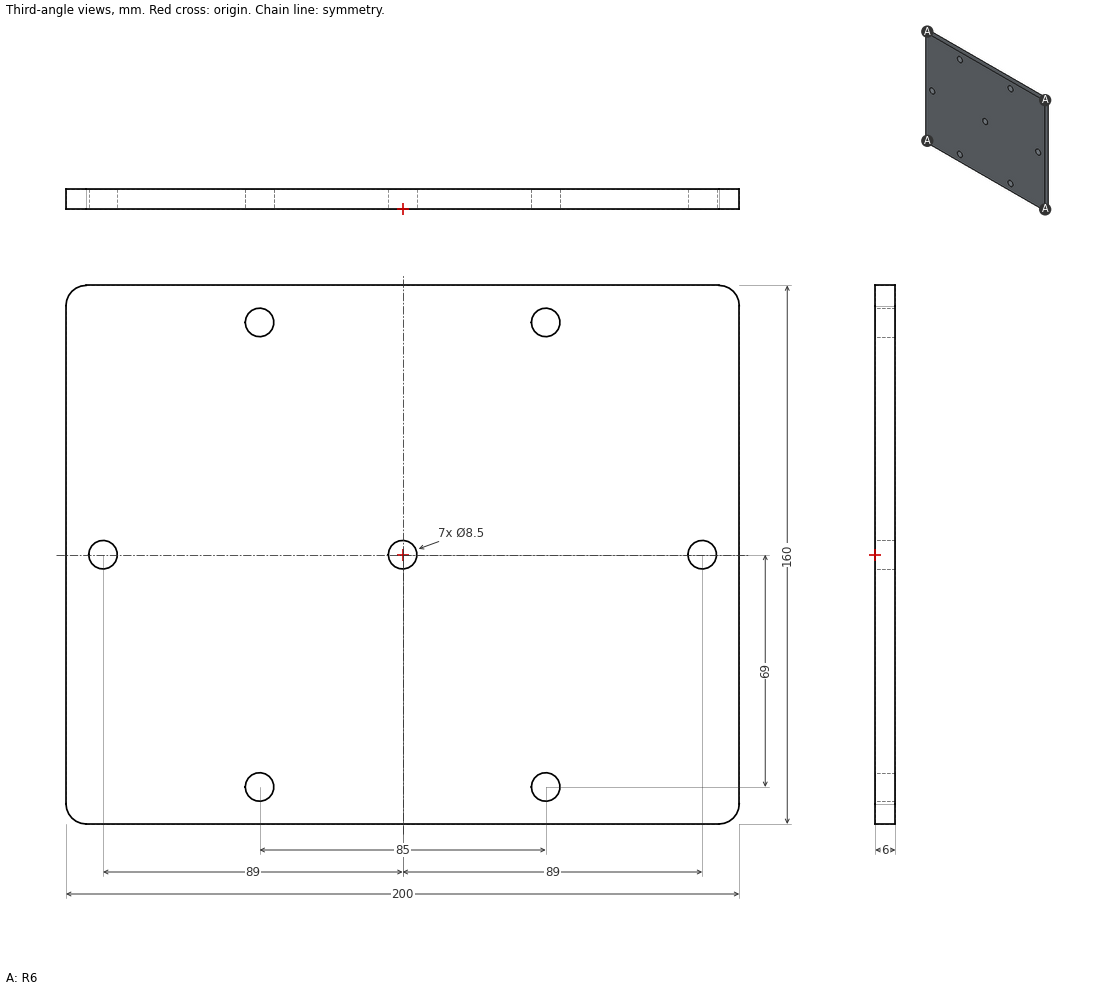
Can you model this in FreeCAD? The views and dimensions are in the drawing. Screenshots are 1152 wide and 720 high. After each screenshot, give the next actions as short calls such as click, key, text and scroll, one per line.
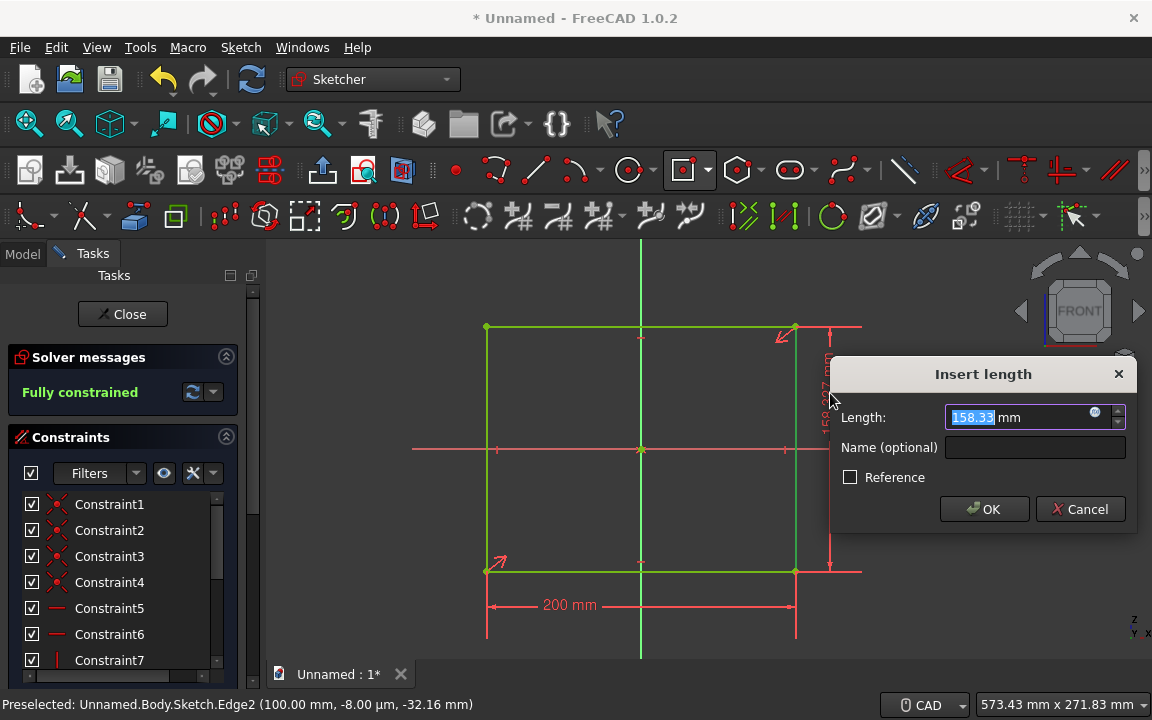
text(160)
key(Return)
key(Escape)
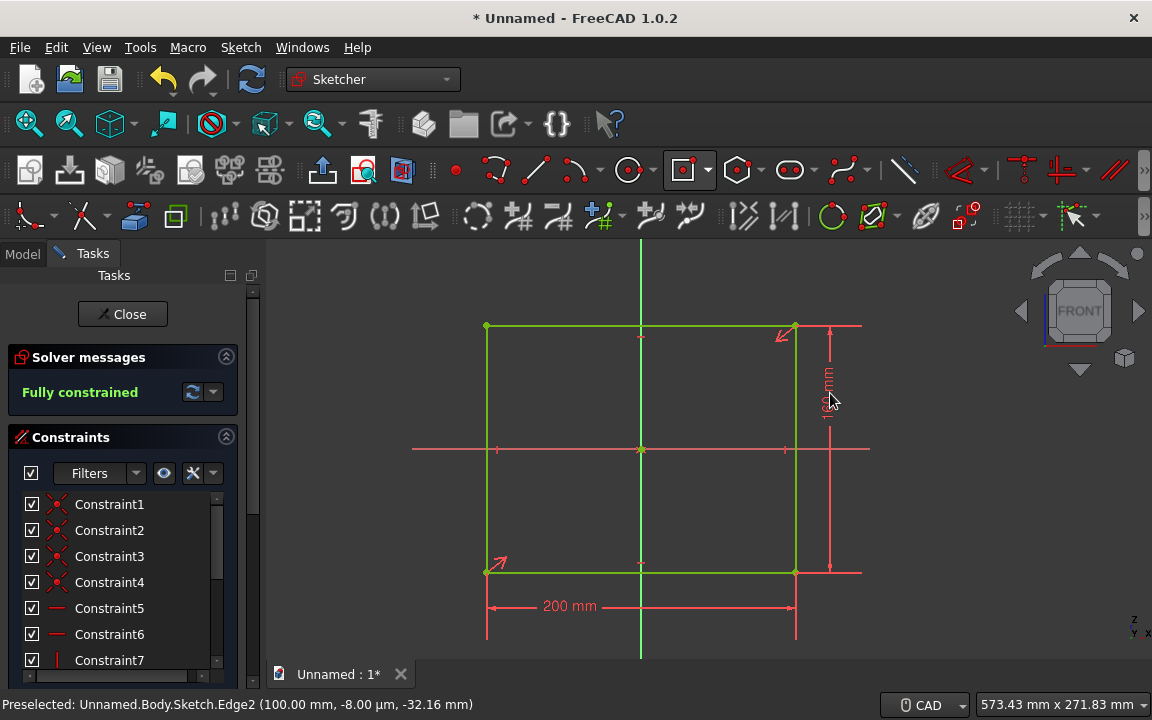
click(123, 314)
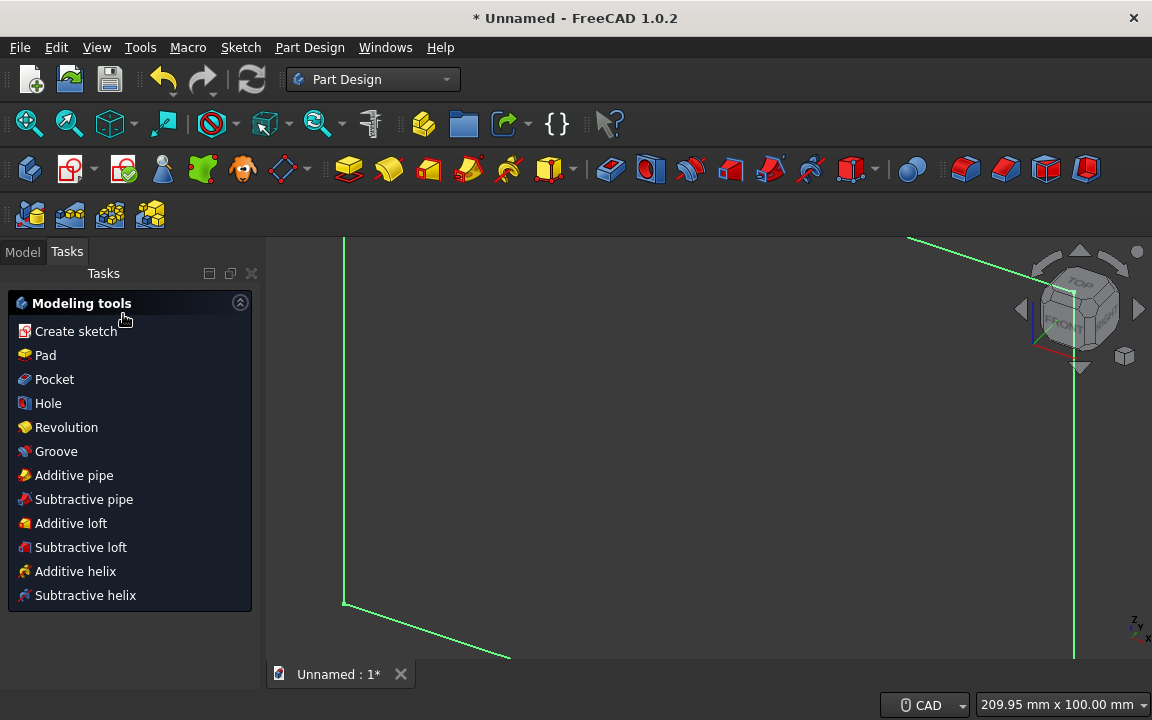
click(350, 170)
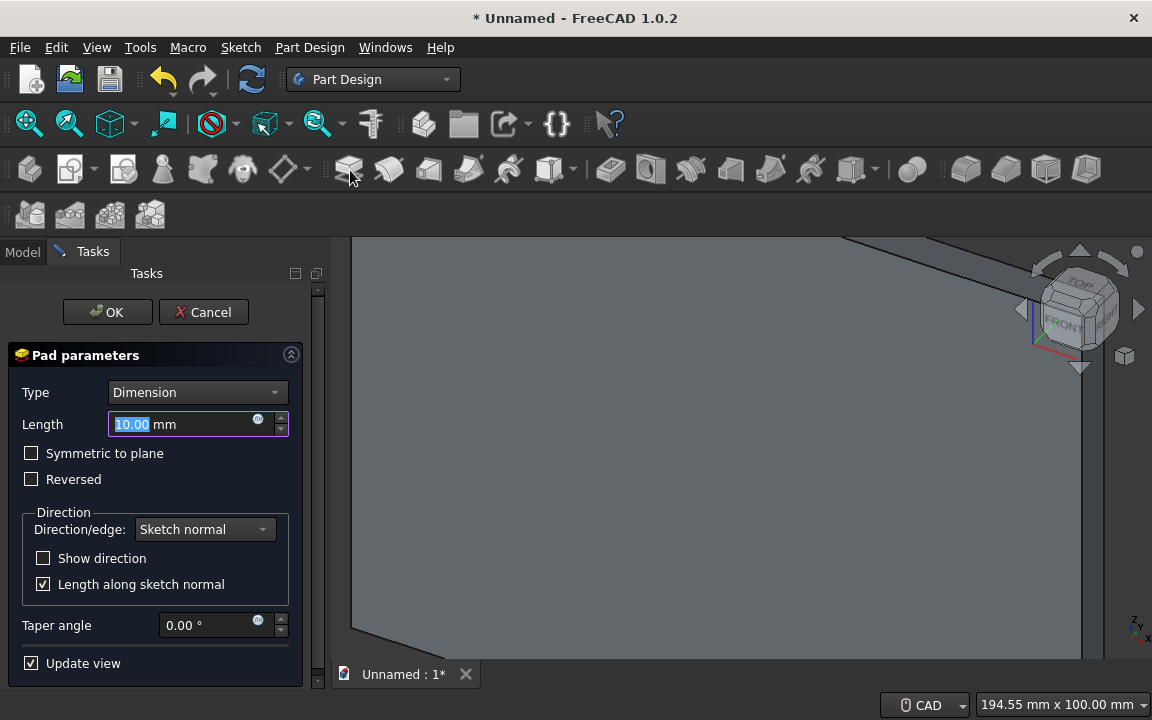
text(6)
key(Tab)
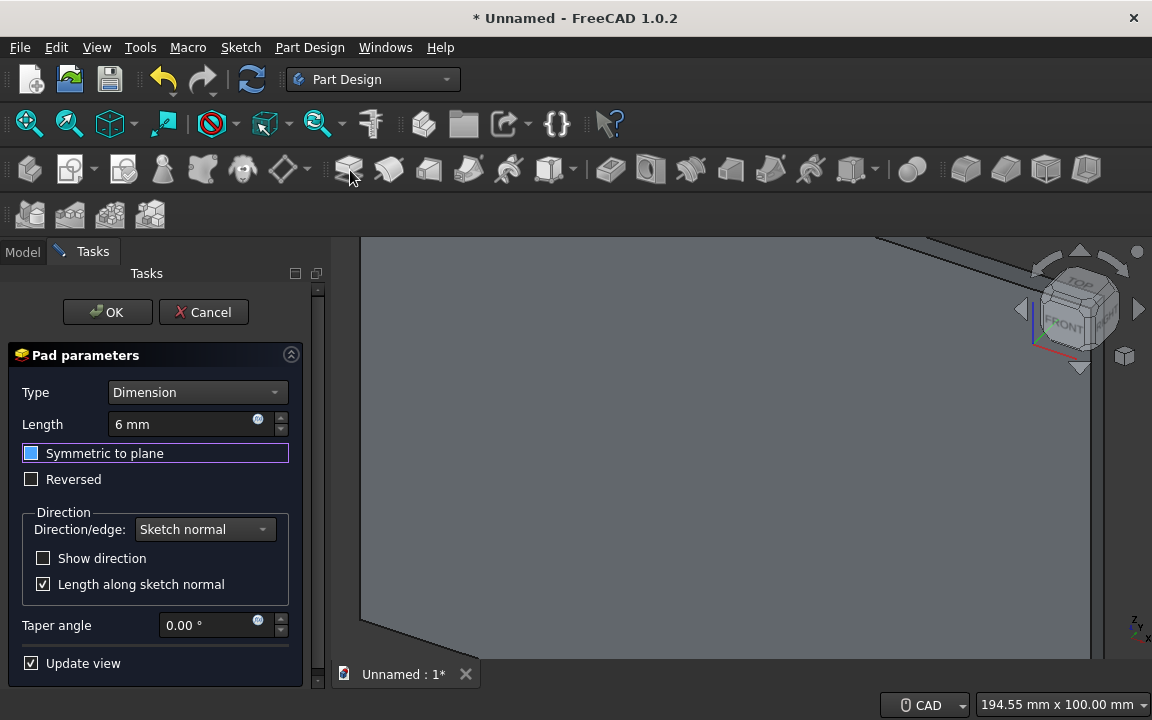
click(30, 479)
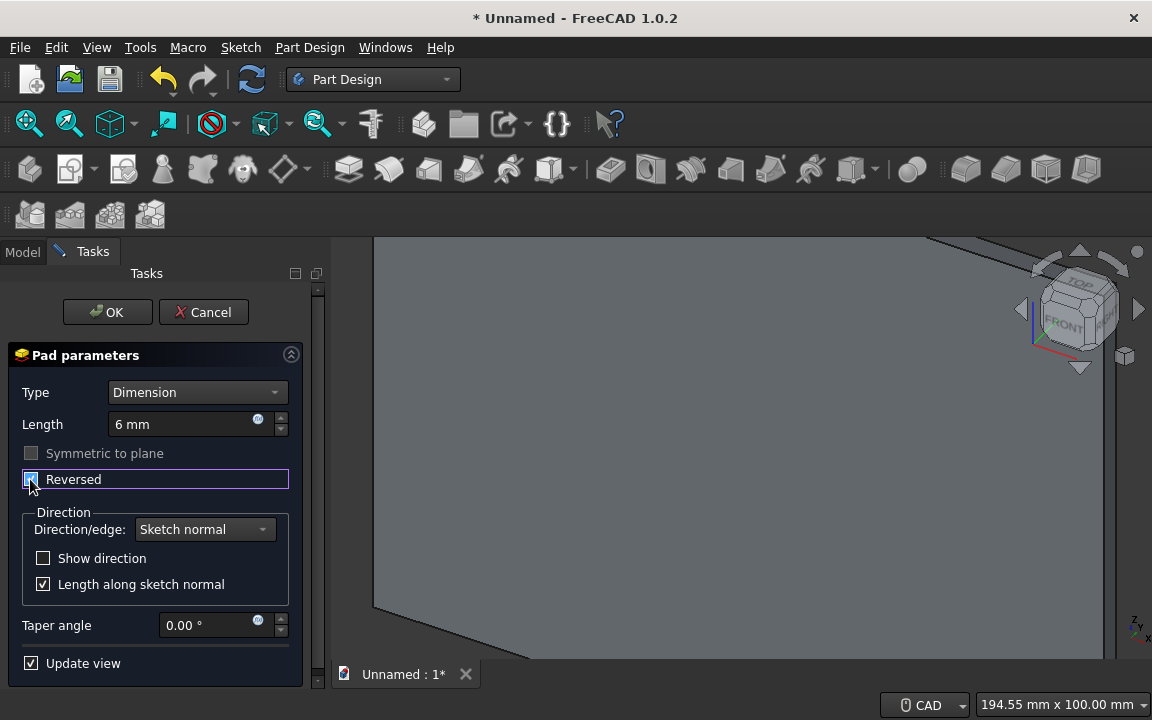
click(108, 312)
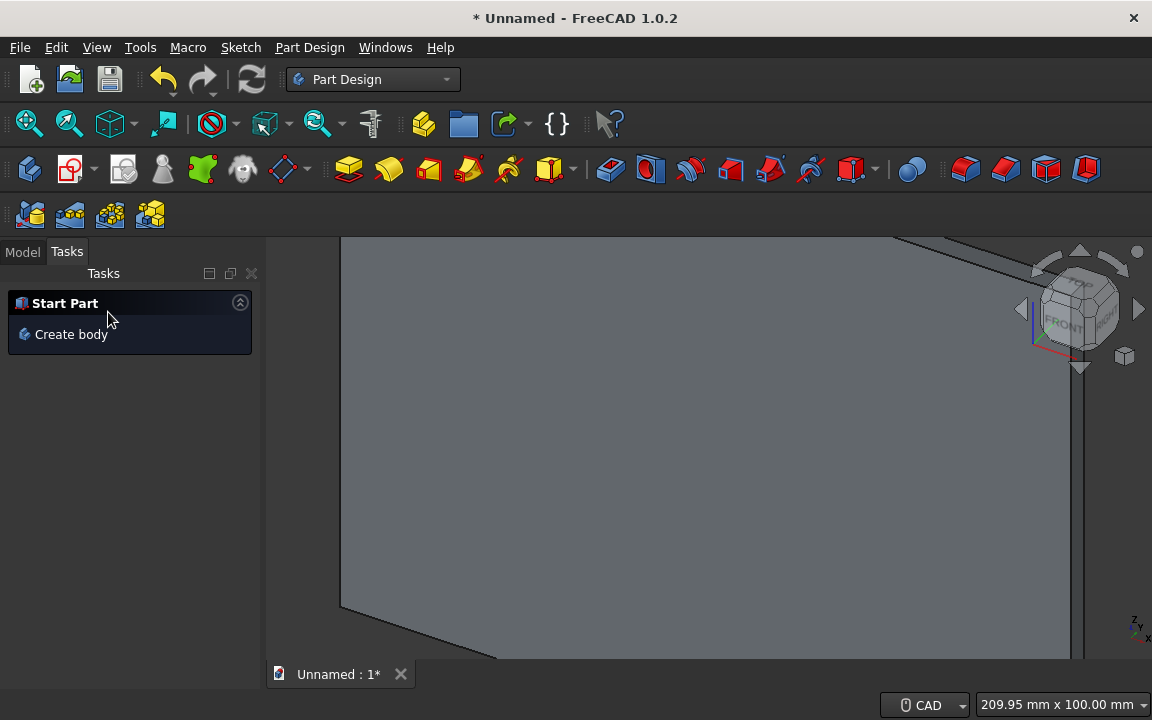
click(30, 124)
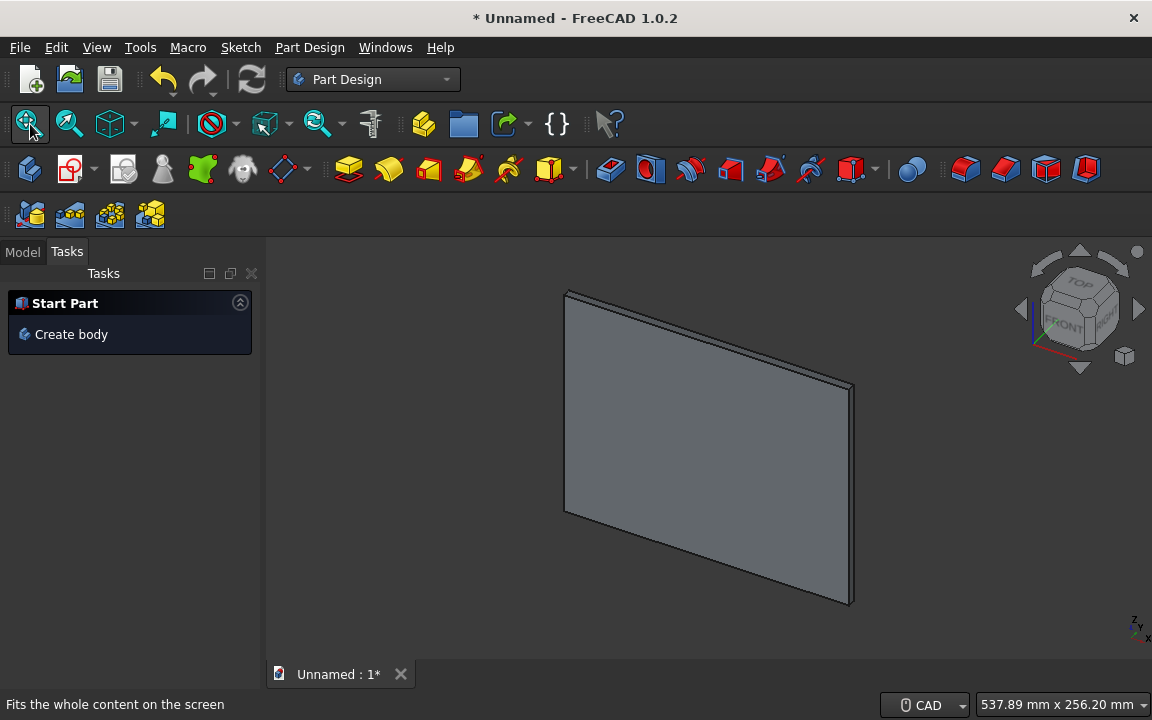
scroll(852, 386, up, 7)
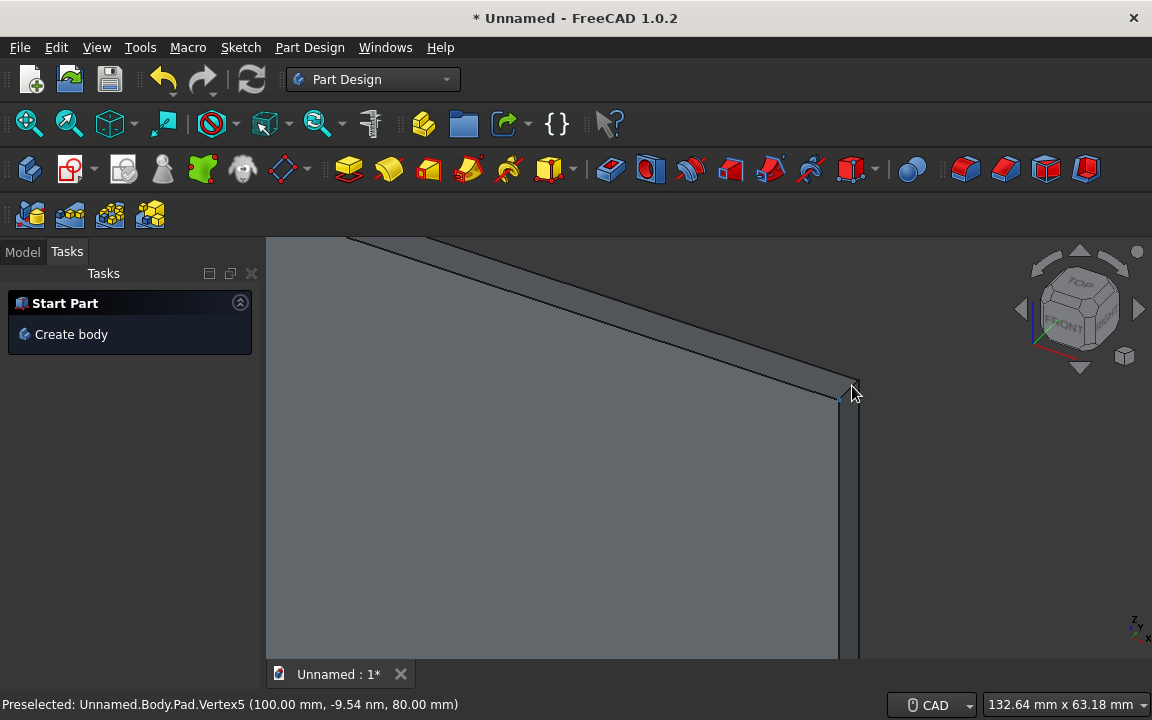
click(849, 389)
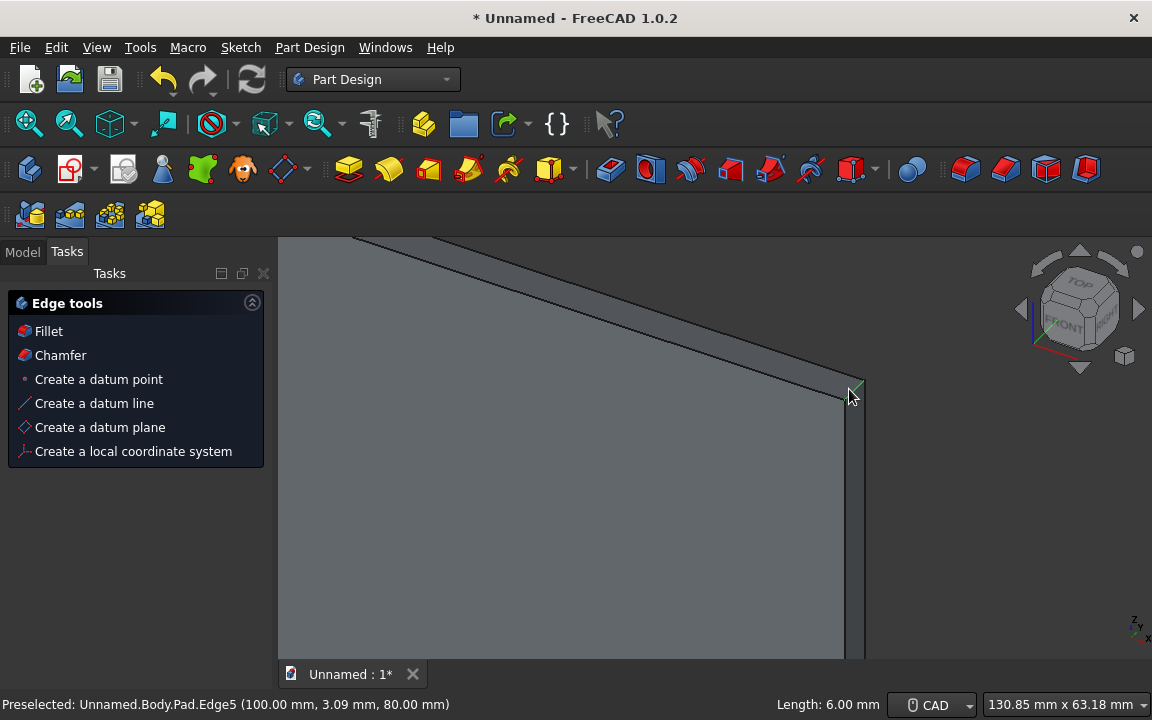
click(30, 124)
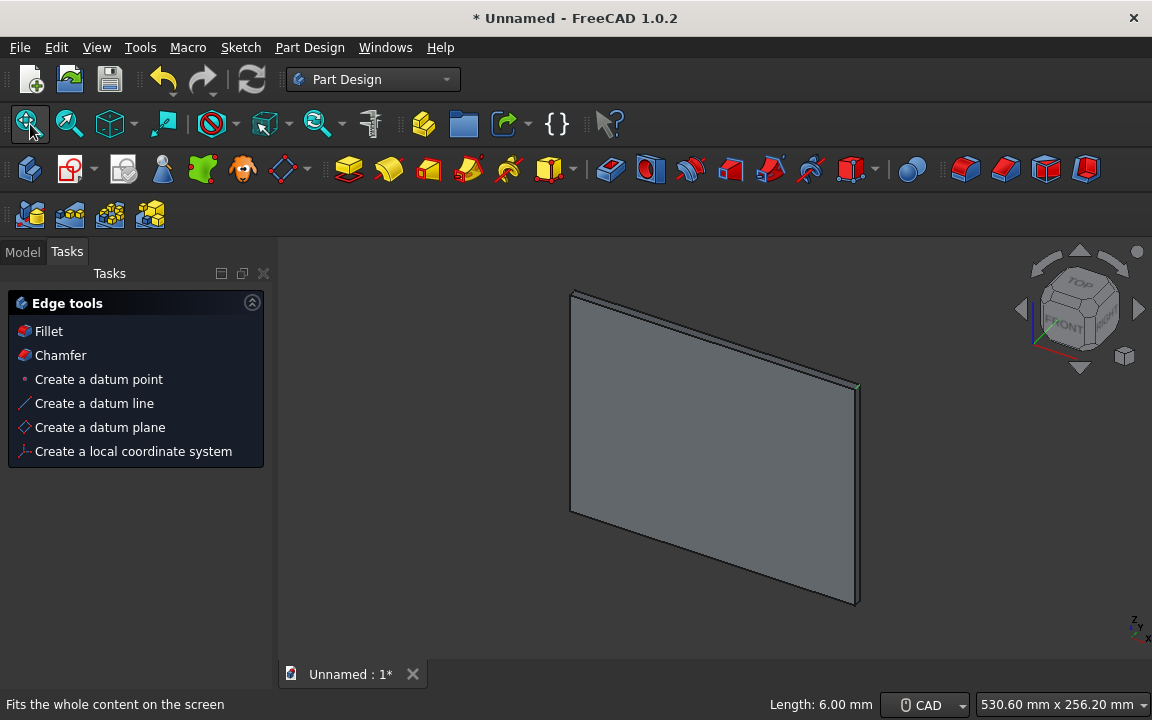
key(0)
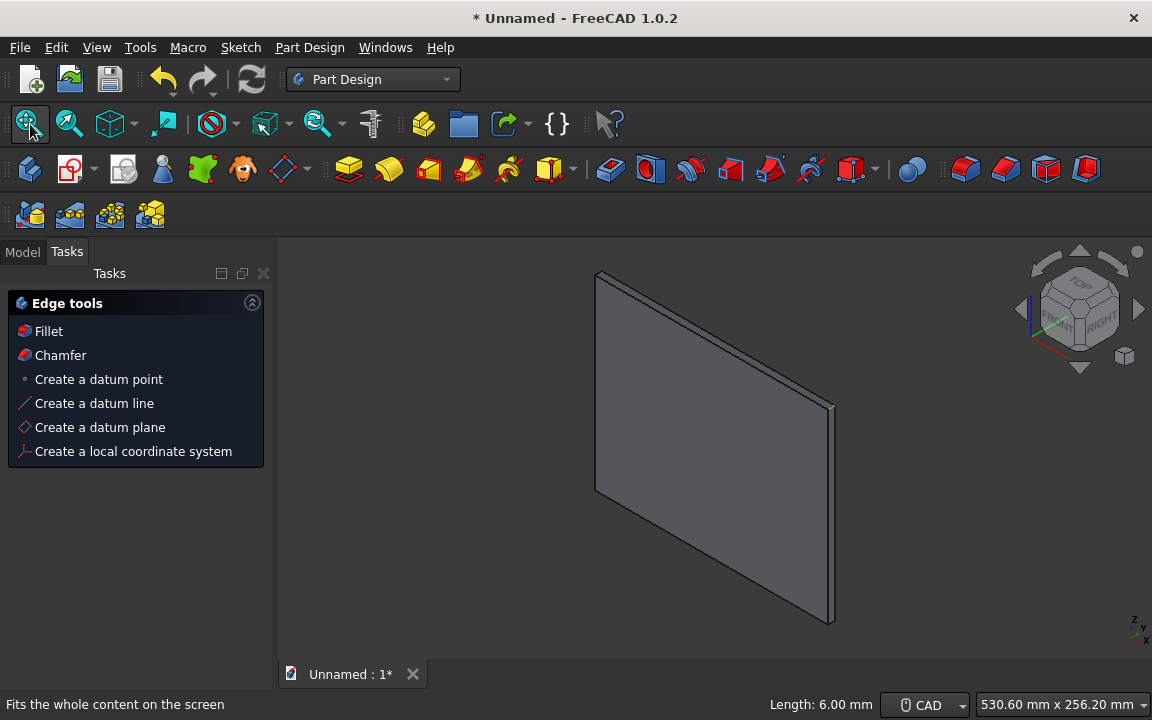
scroll(599, 272, up, 7)